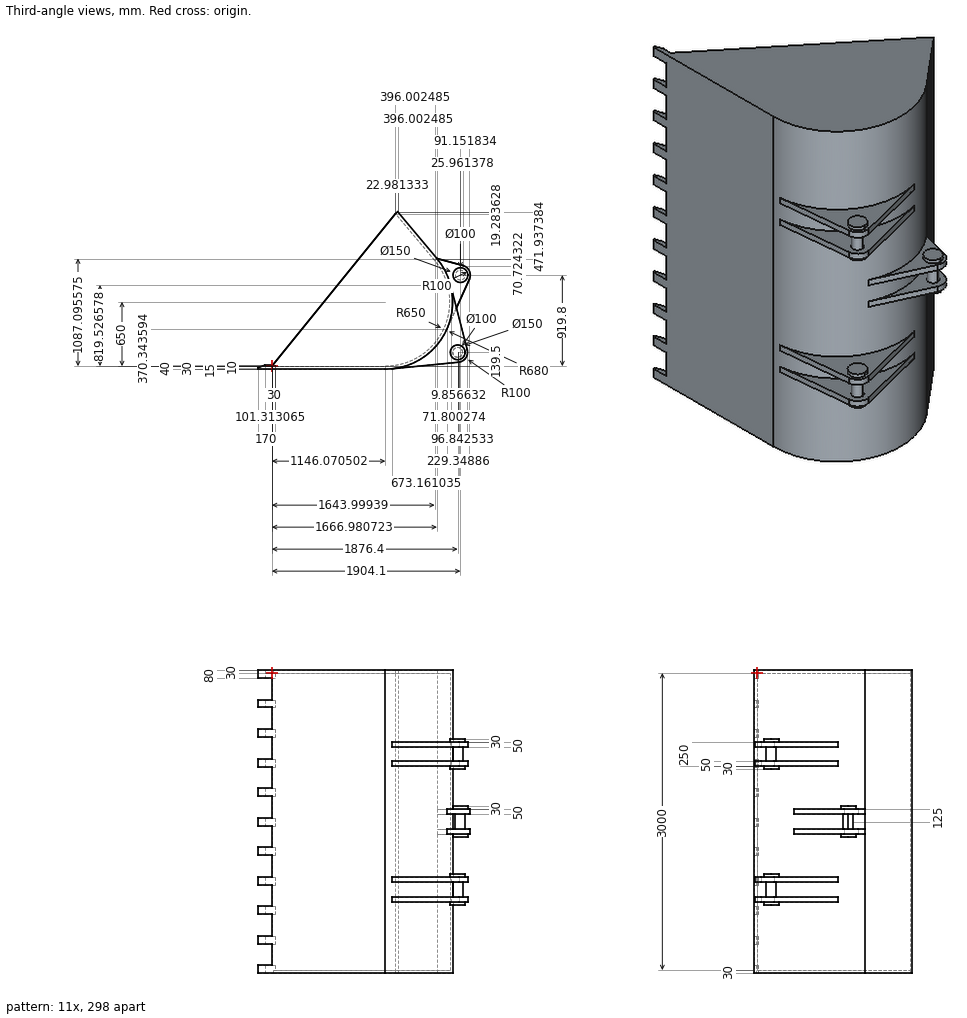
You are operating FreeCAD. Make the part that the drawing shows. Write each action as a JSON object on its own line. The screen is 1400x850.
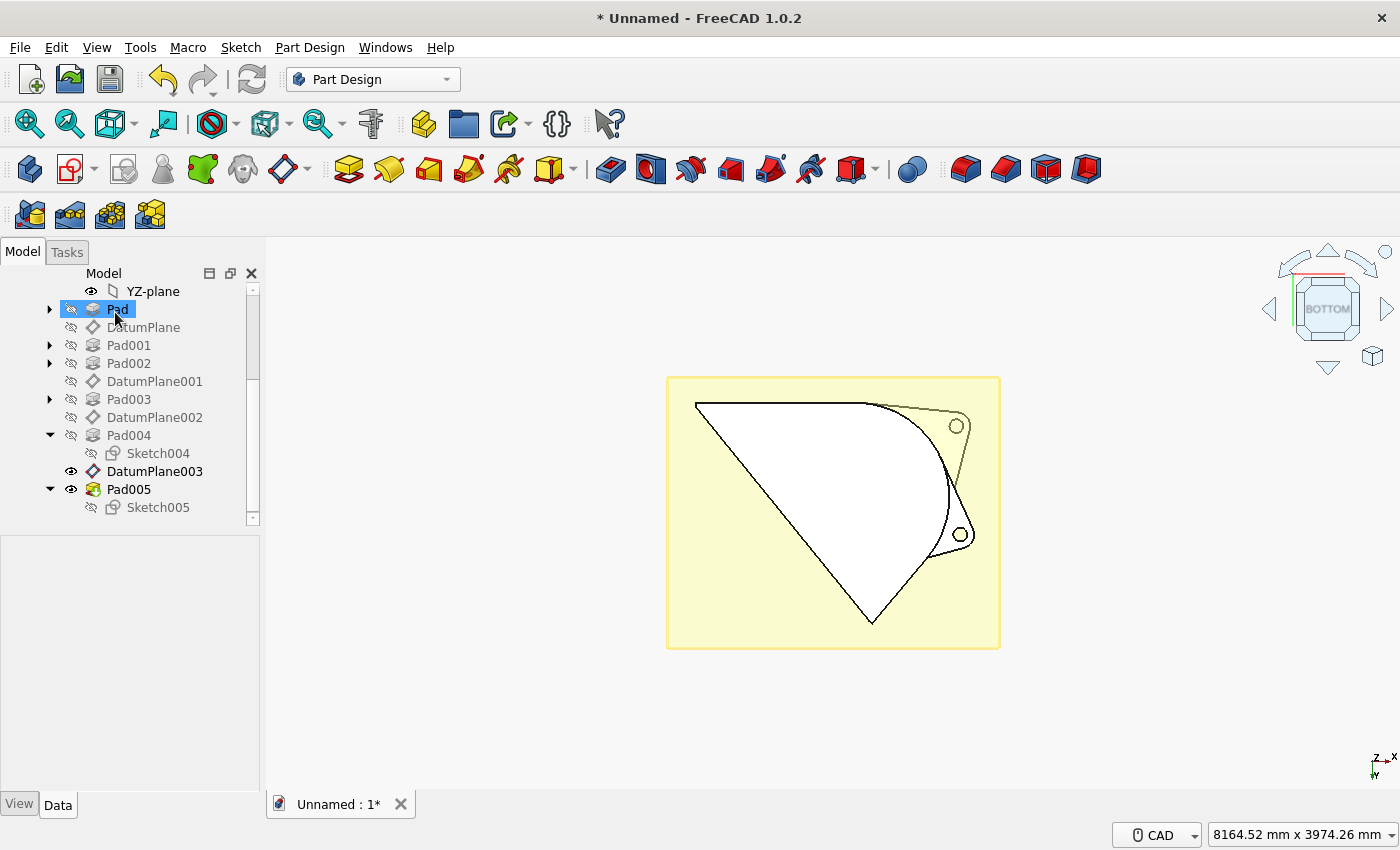
{"action": "left_click", "coordinate": [116, 471]}
{"action": "key", "text": "space"}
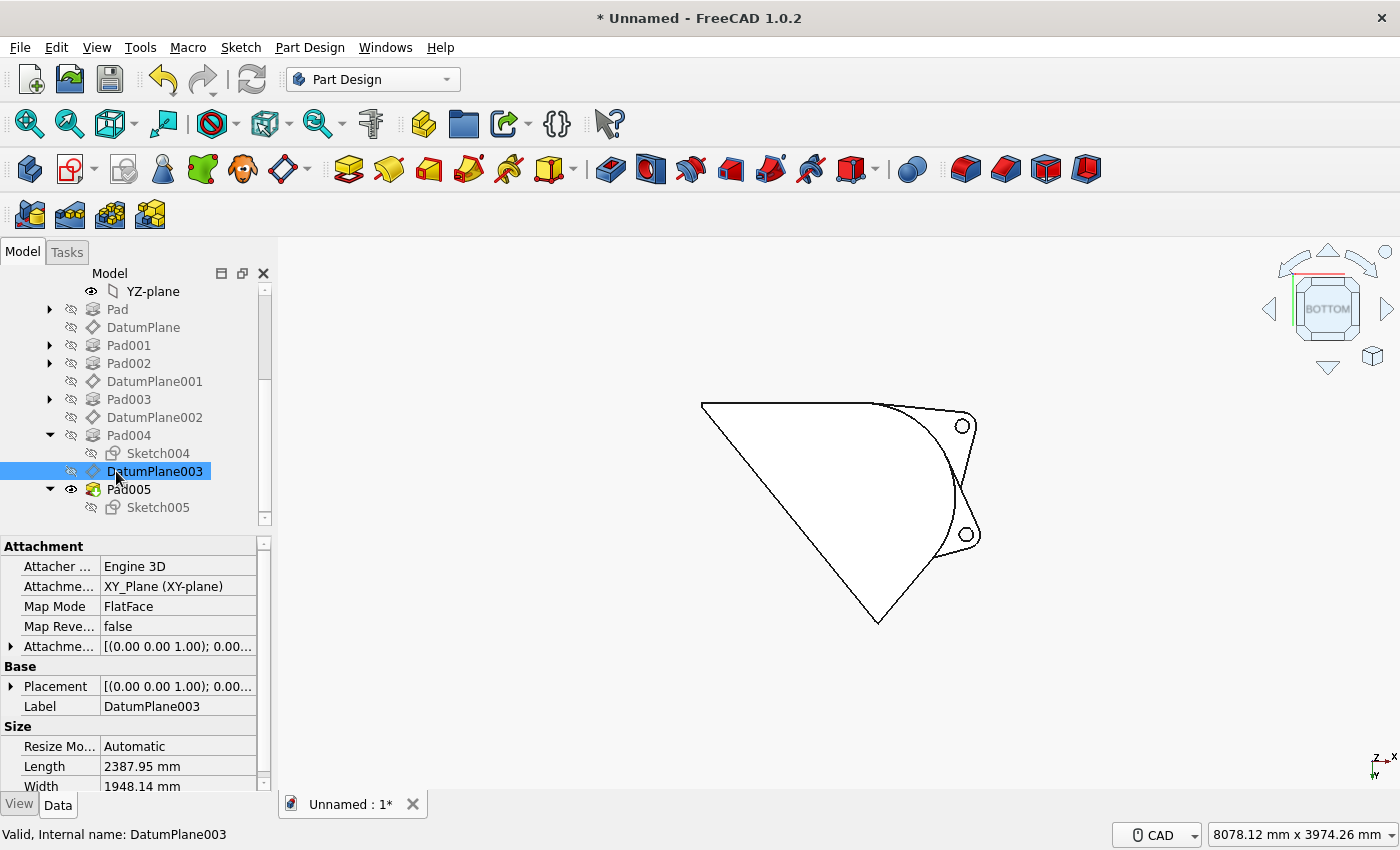
{"action": "key", "text": "v f"}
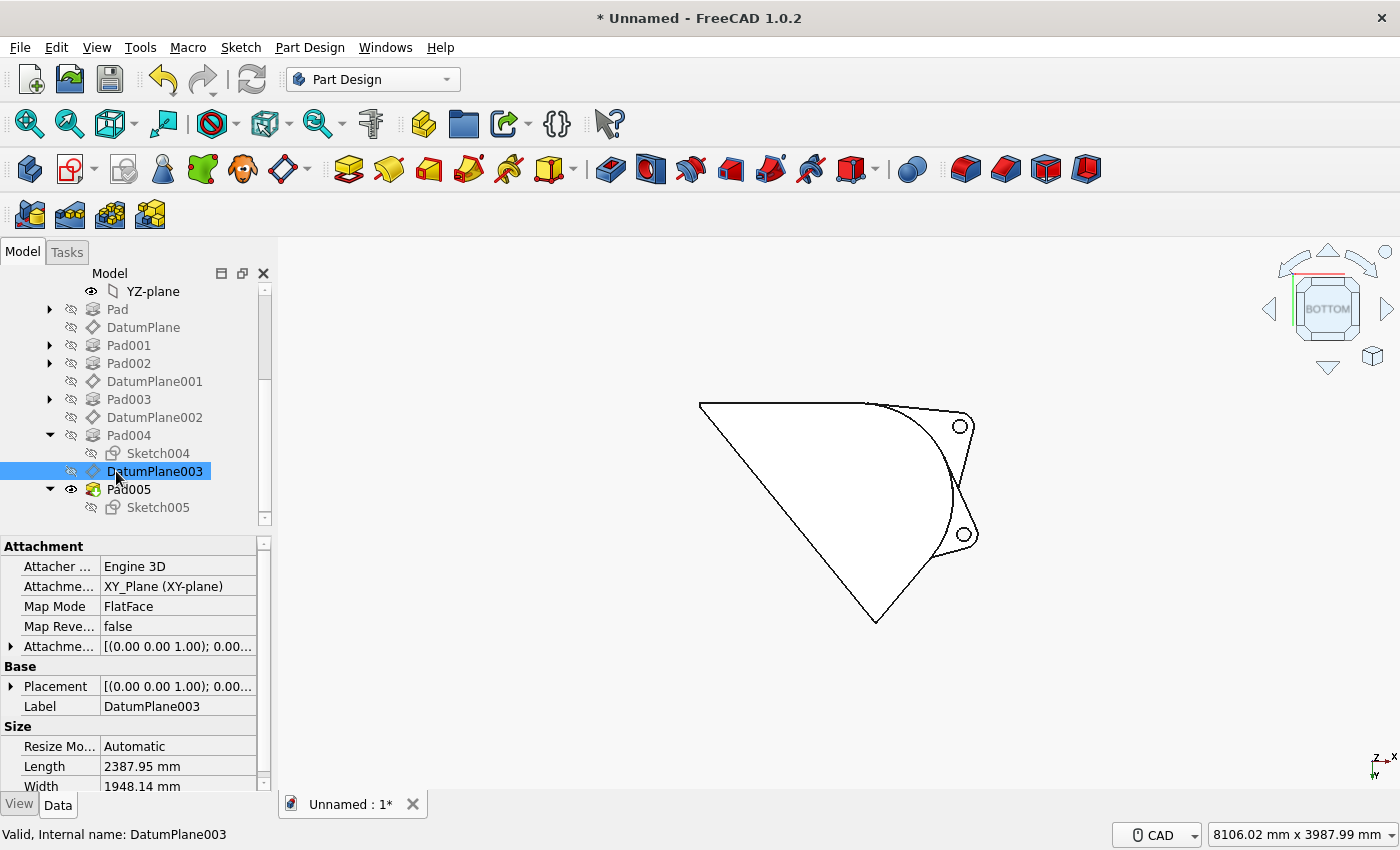
{"action": "key", "text": "0"}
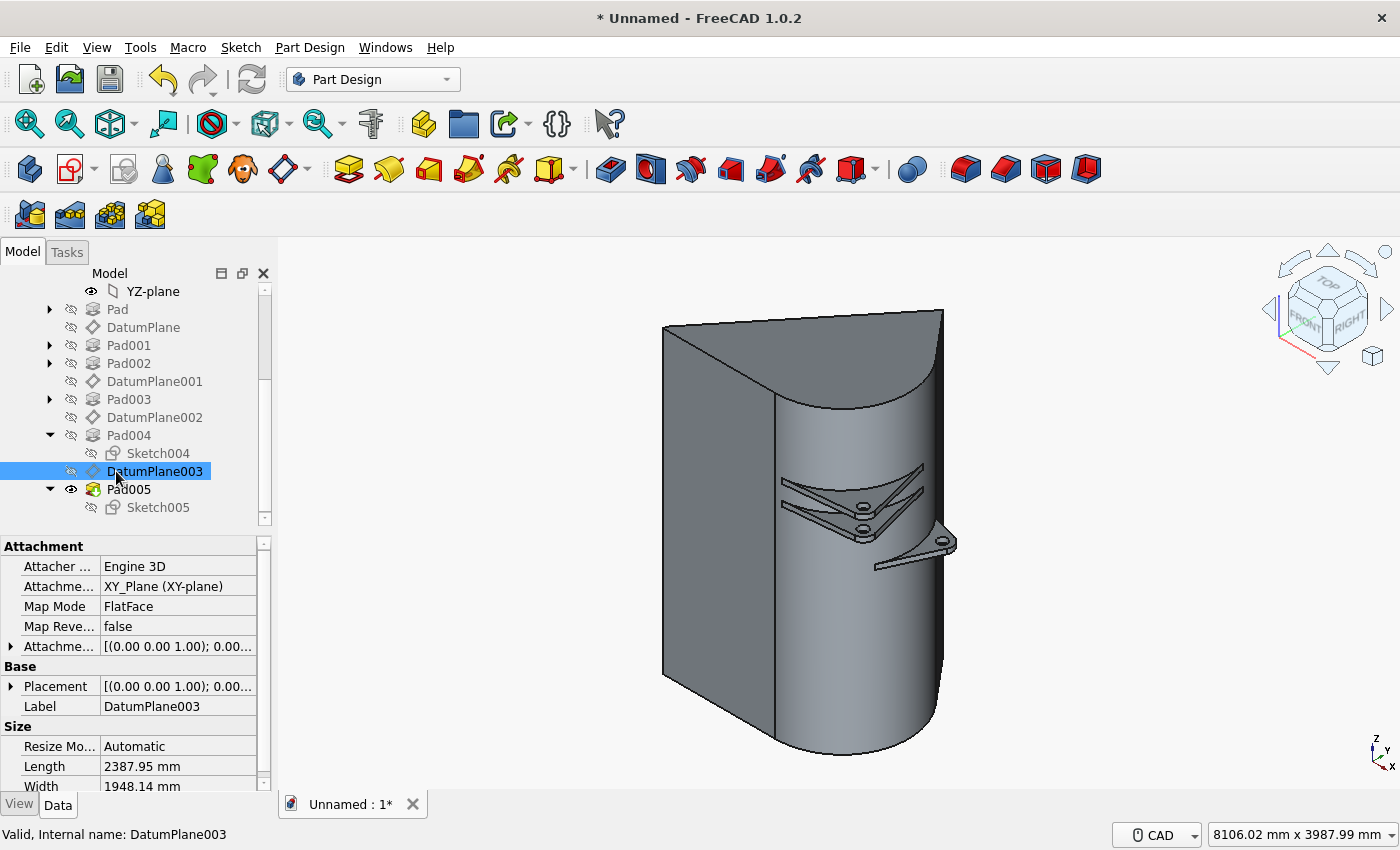
{"action": "left_click", "coordinate": [871, 494]}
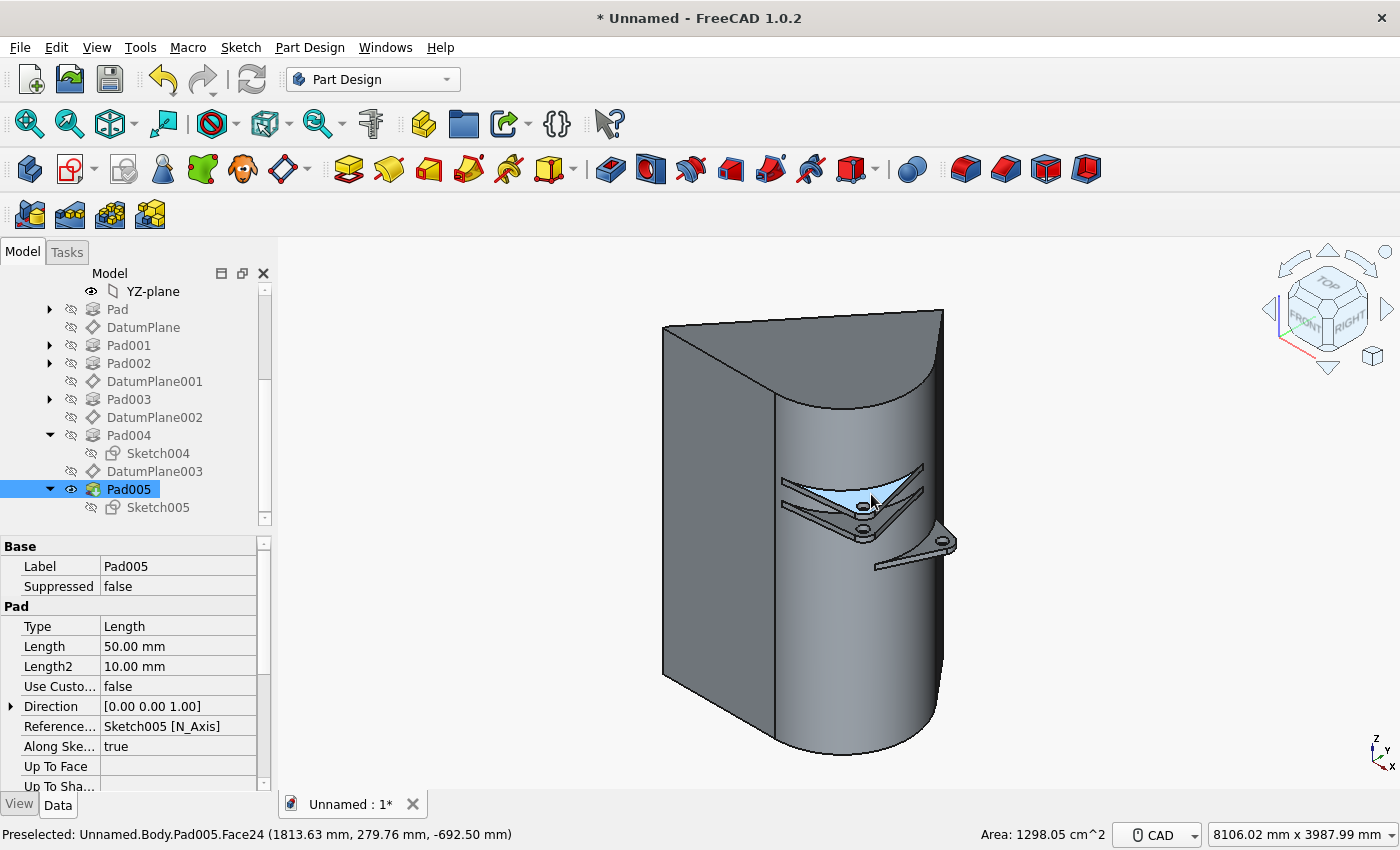
{"action": "left_click", "coordinate": [70, 170]}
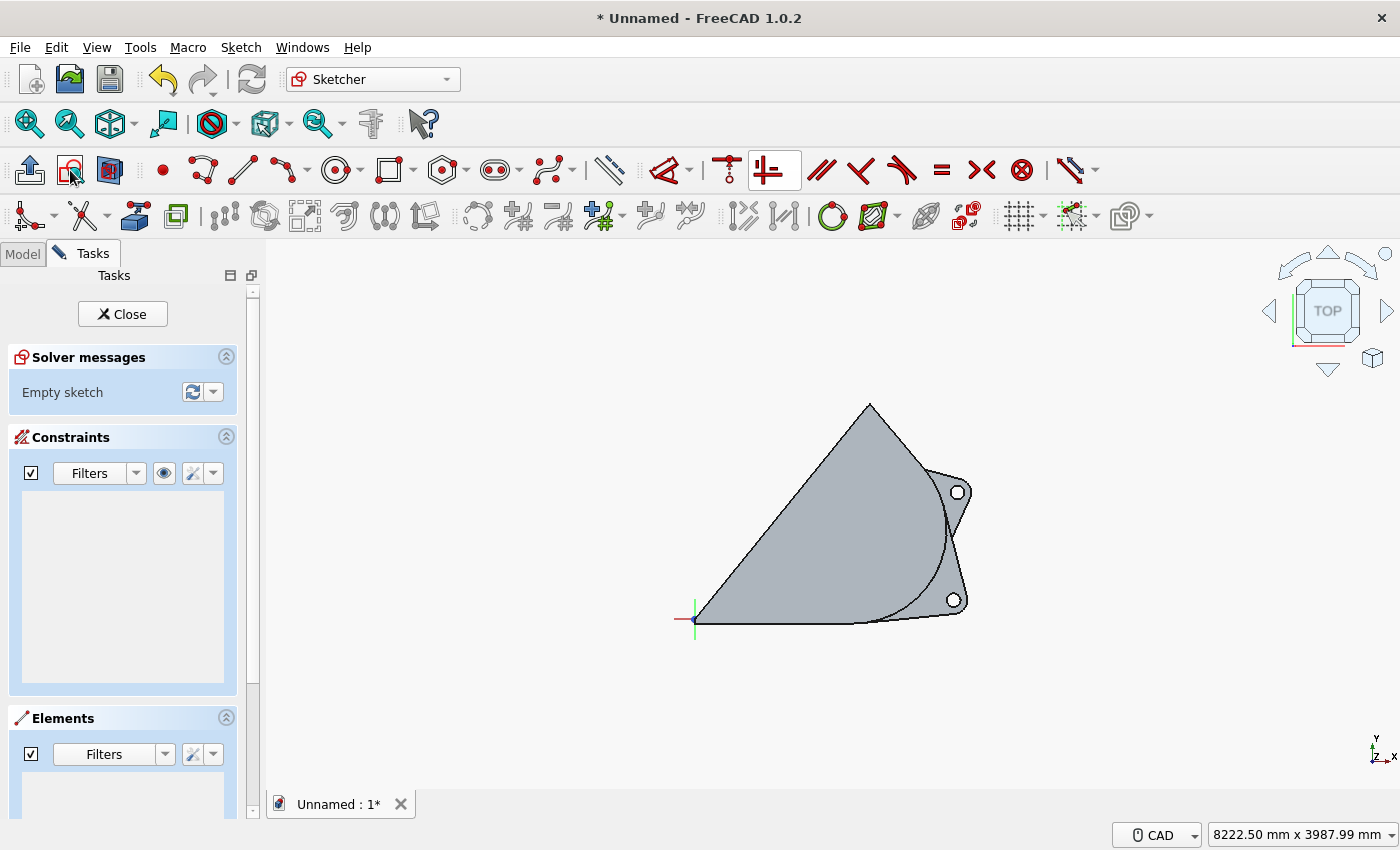
{"action": "scroll", "coordinate": [964, 605], "scroll_direction": "up", "scroll_amount": 15}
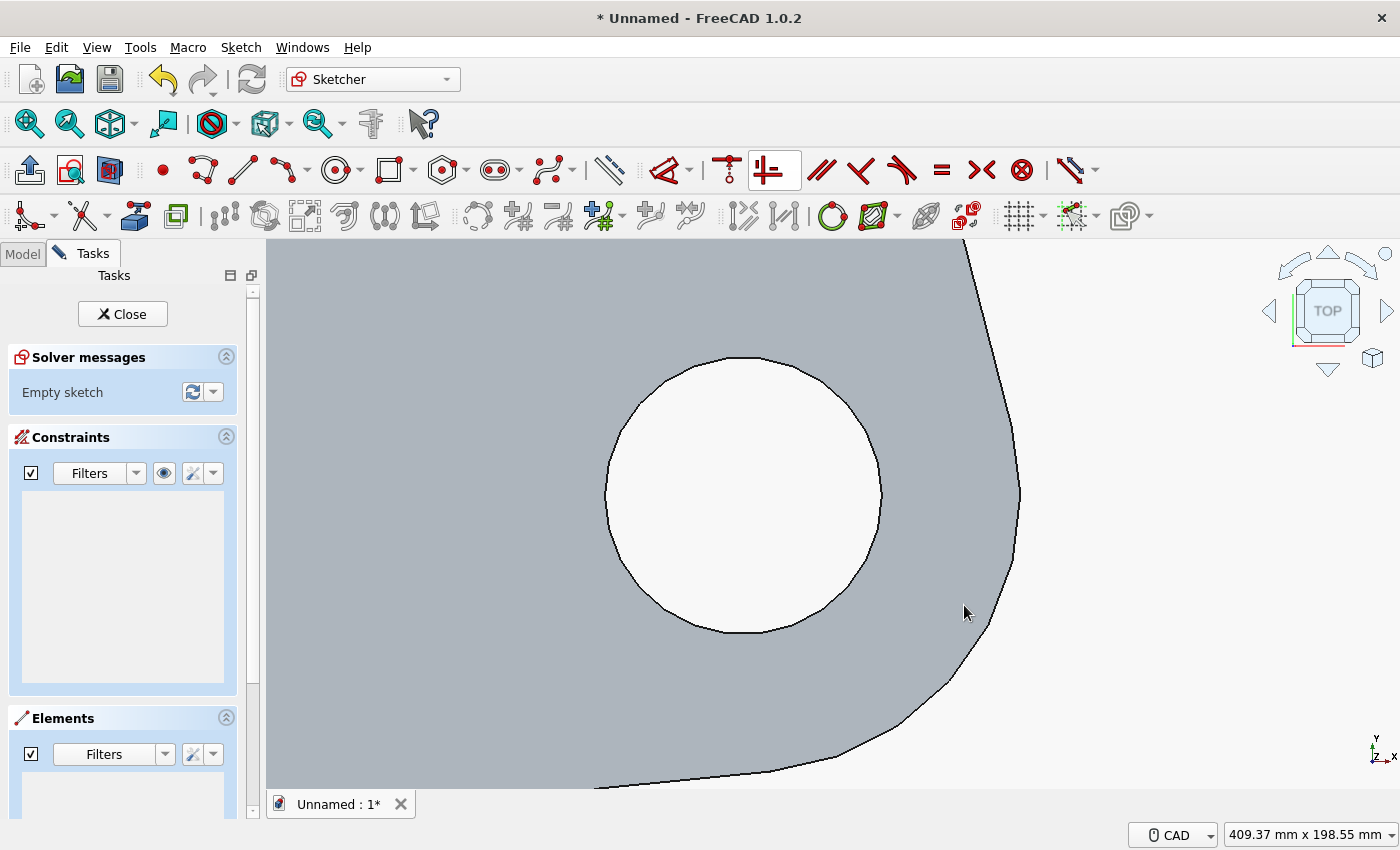
{"action": "left_click", "coordinate": [336, 170]}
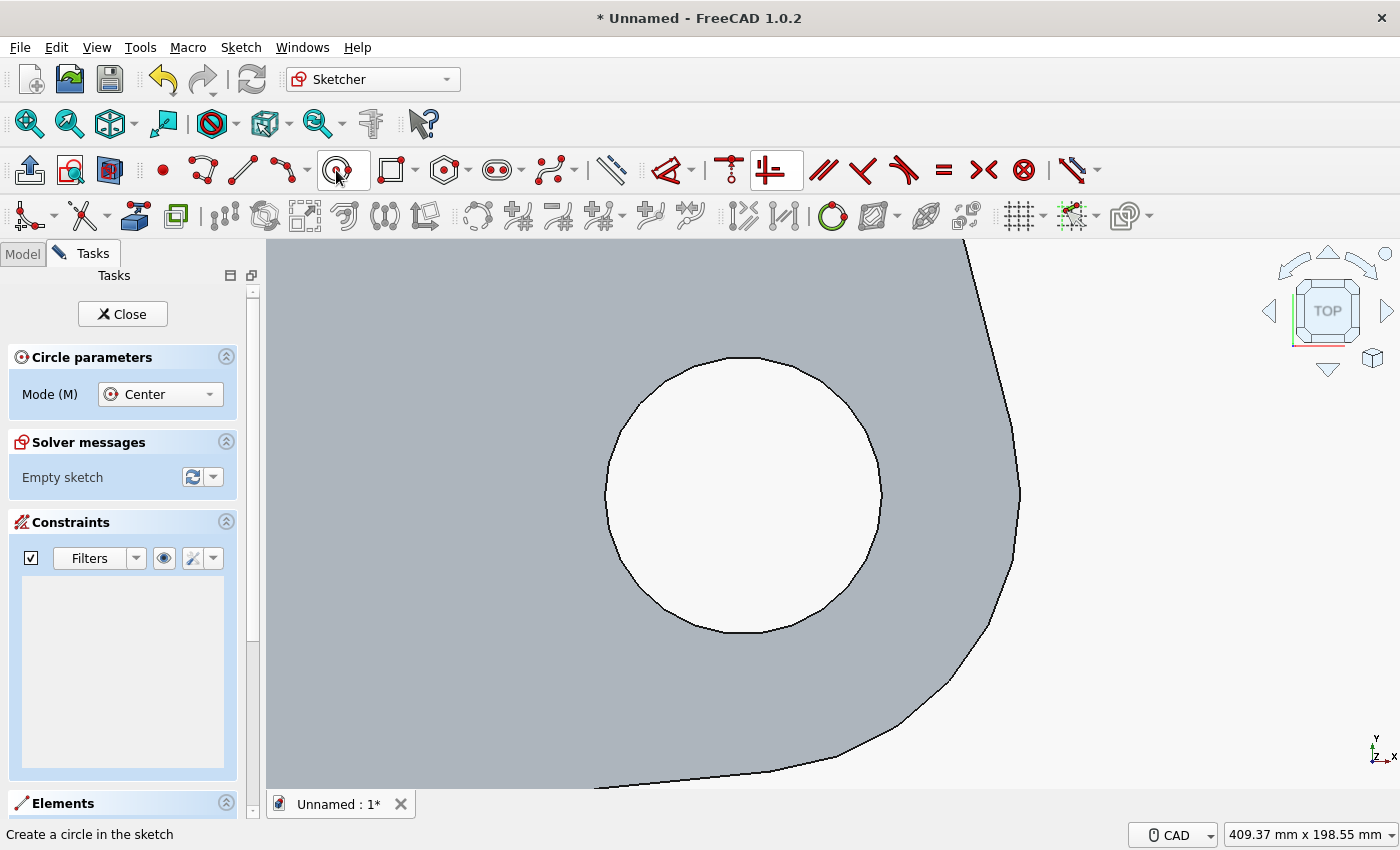
{"action": "left_click", "coordinate": [743, 496]}
{"action": "left_click", "coordinate": [841, 398]}
{"action": "key", "text": "Escape"}